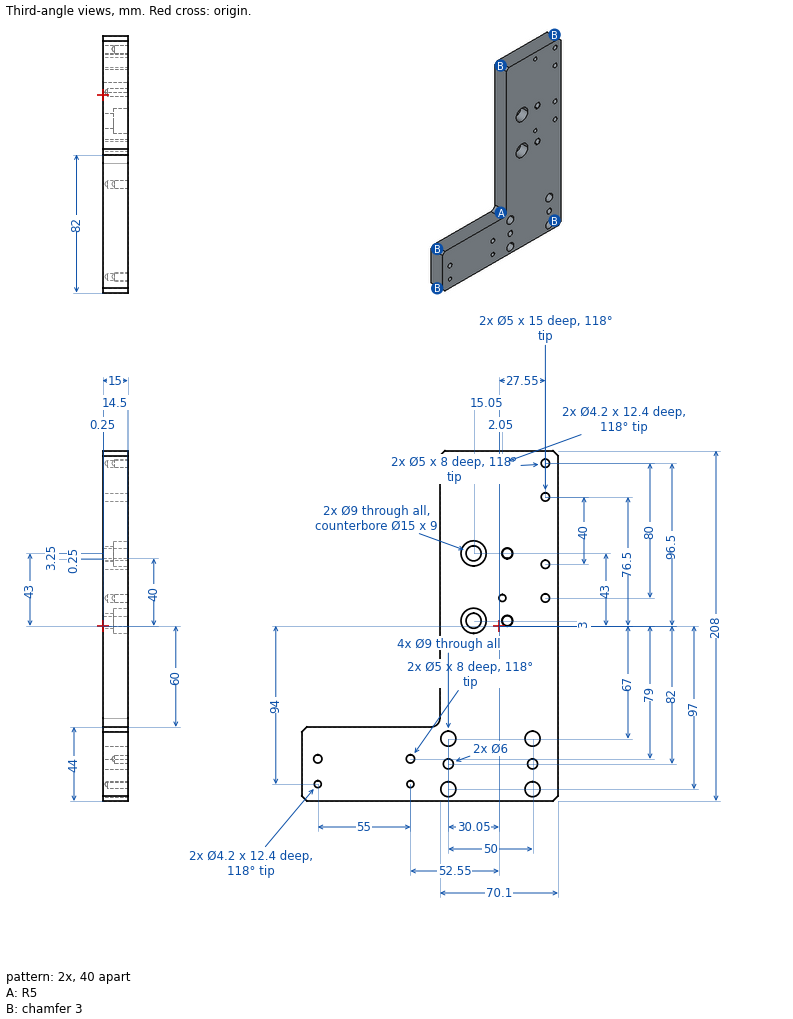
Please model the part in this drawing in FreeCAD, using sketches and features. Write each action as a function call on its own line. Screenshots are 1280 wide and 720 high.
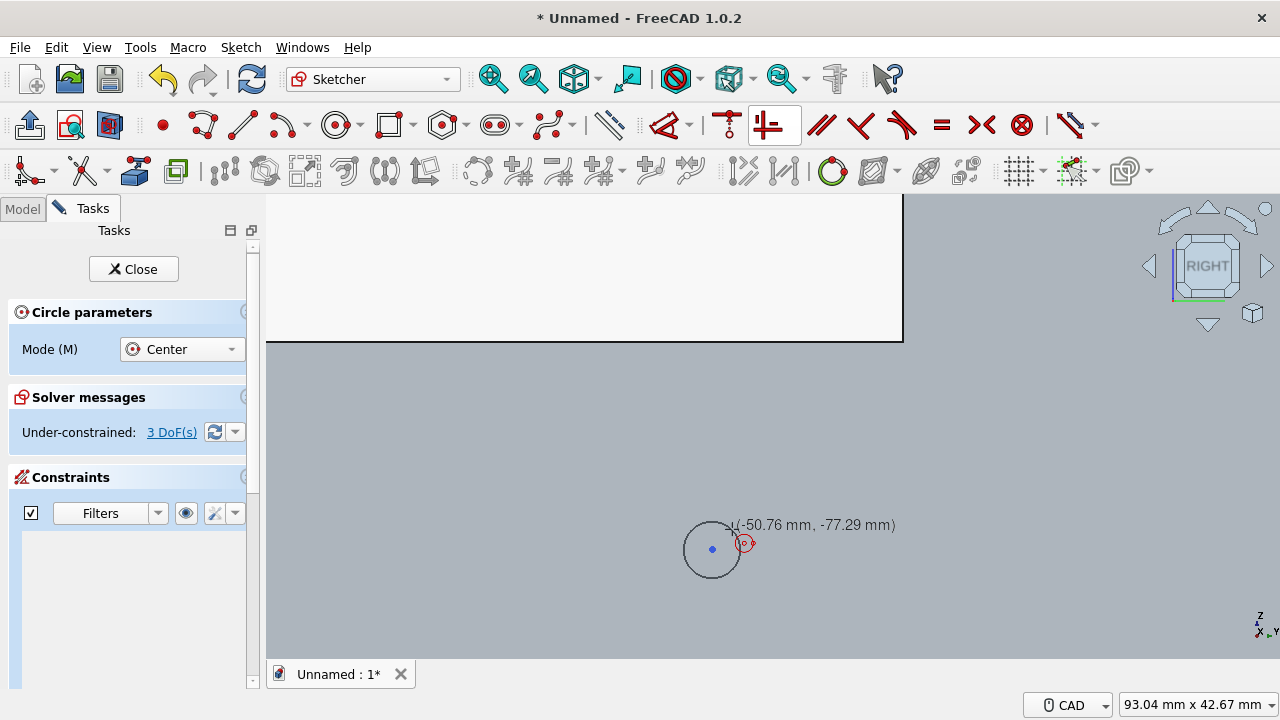
scroll(713, 554, down, 6)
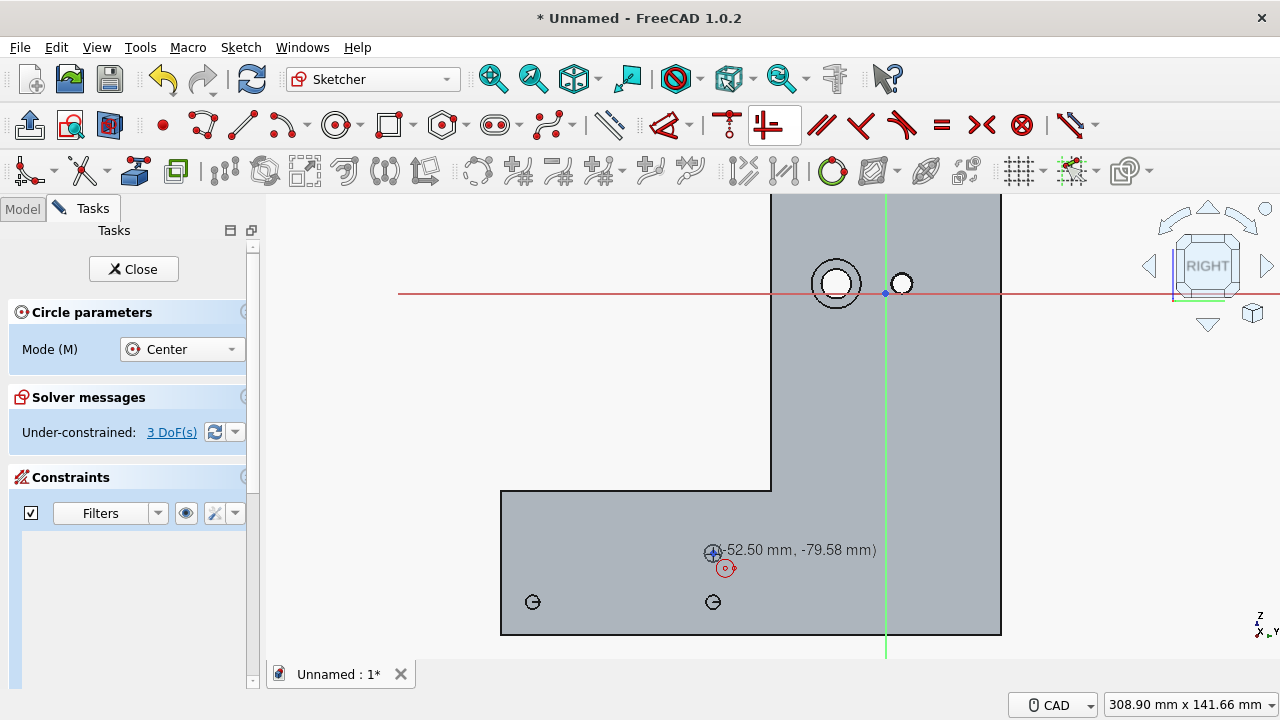
scroll(533, 553, up, 6)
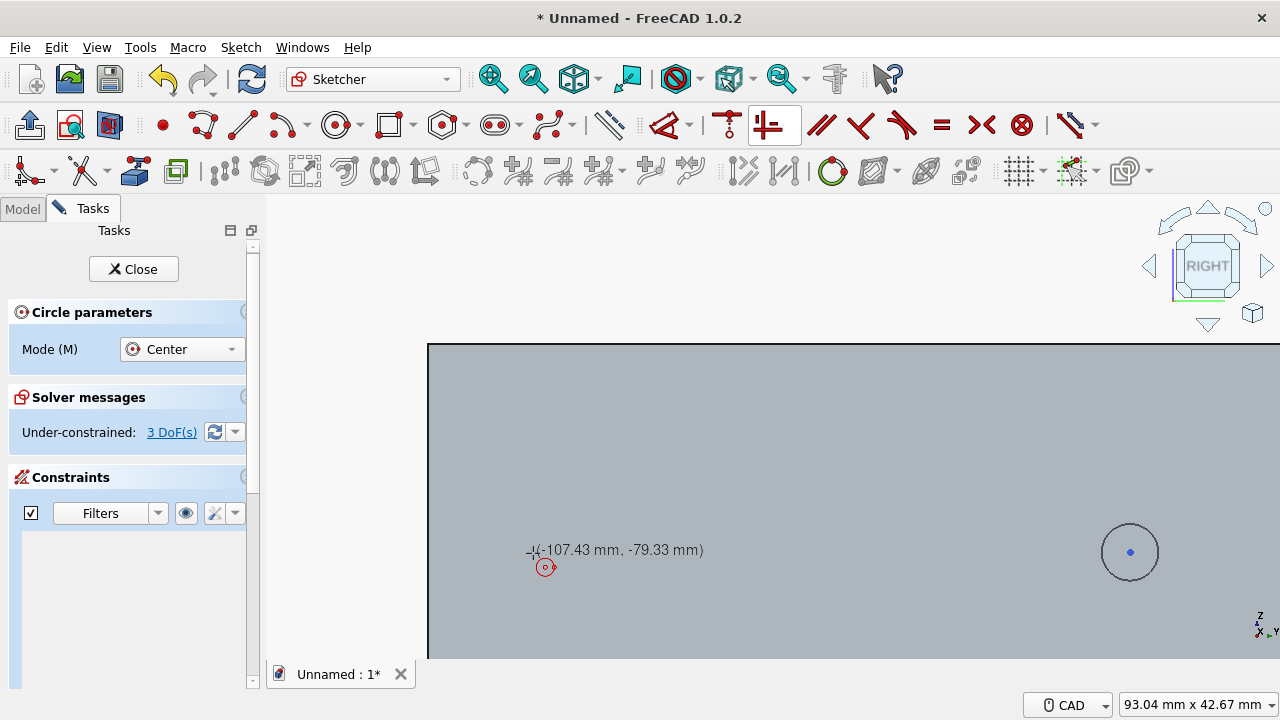
click(531, 551)
click(550, 532)
key(Escape)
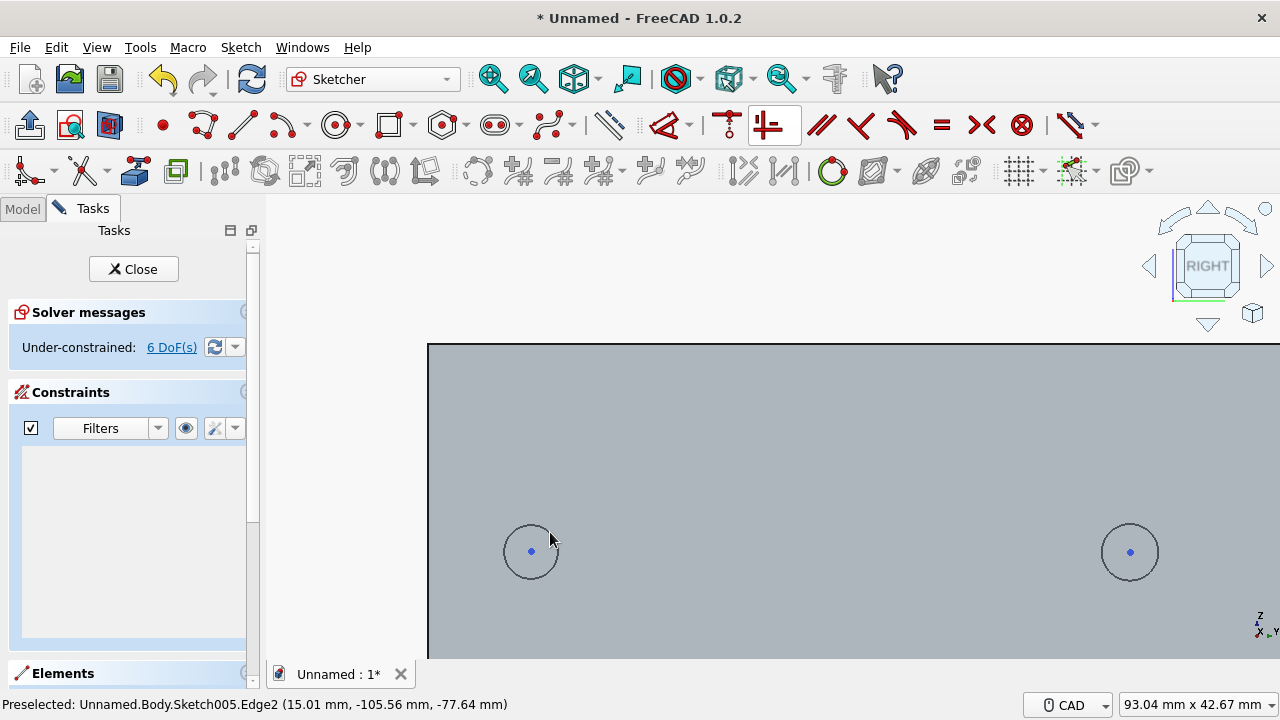
click(1110, 532)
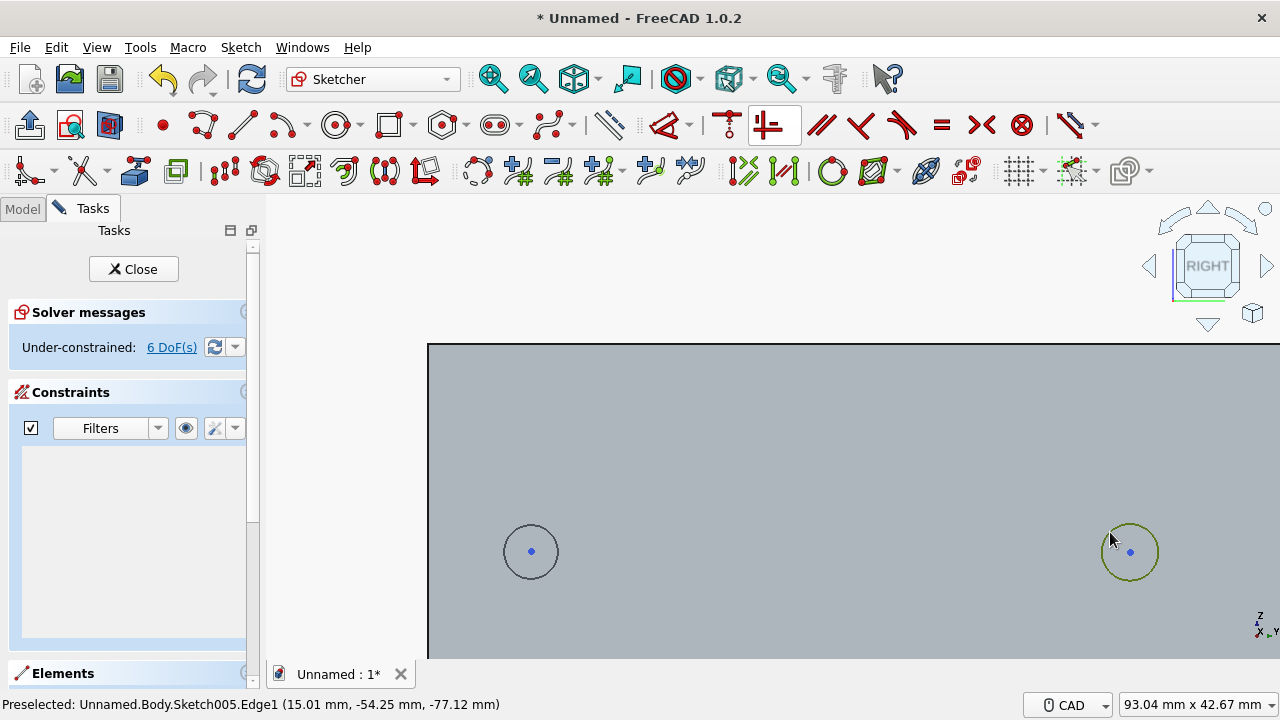
click(550, 533)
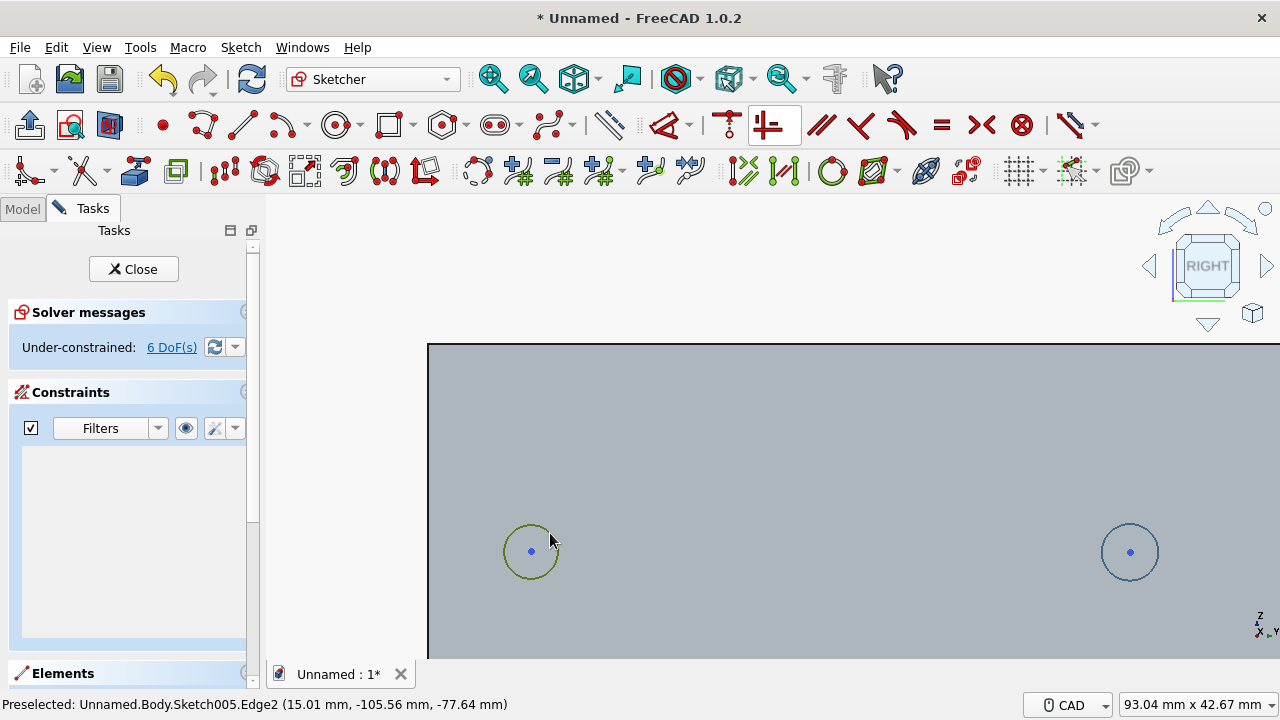
click(942, 126)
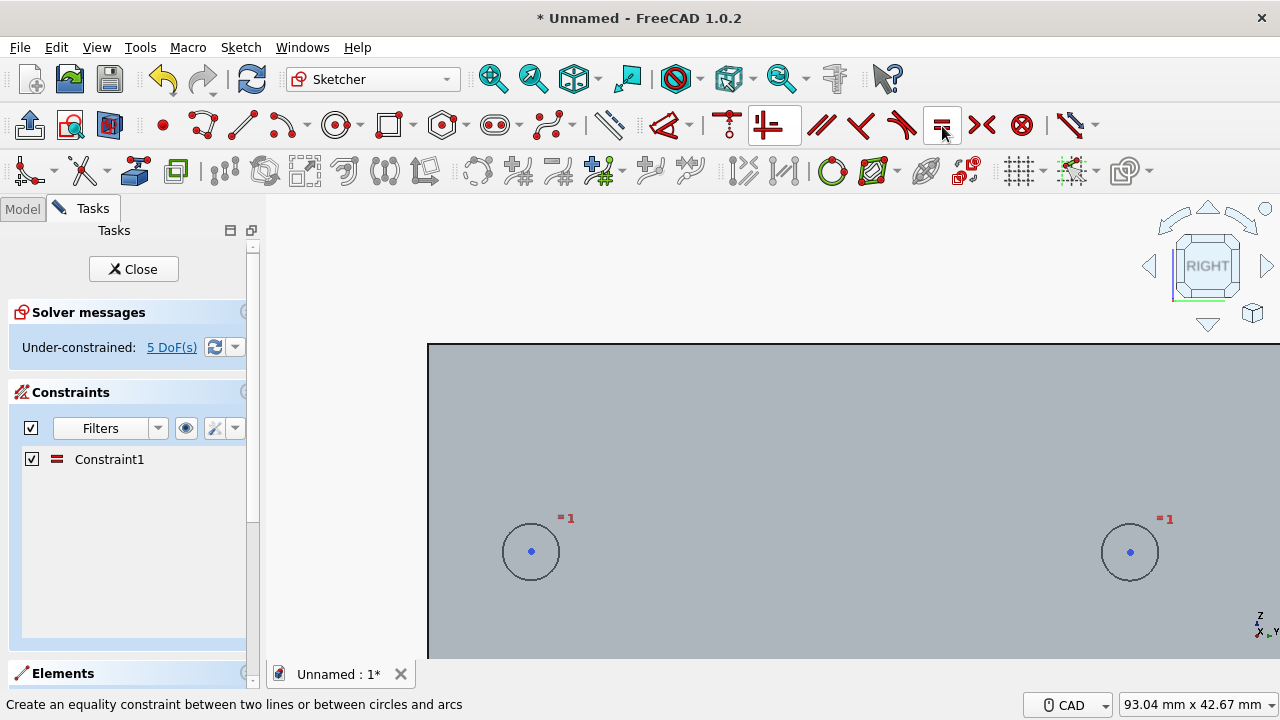
scroll(533, 553, down, 6)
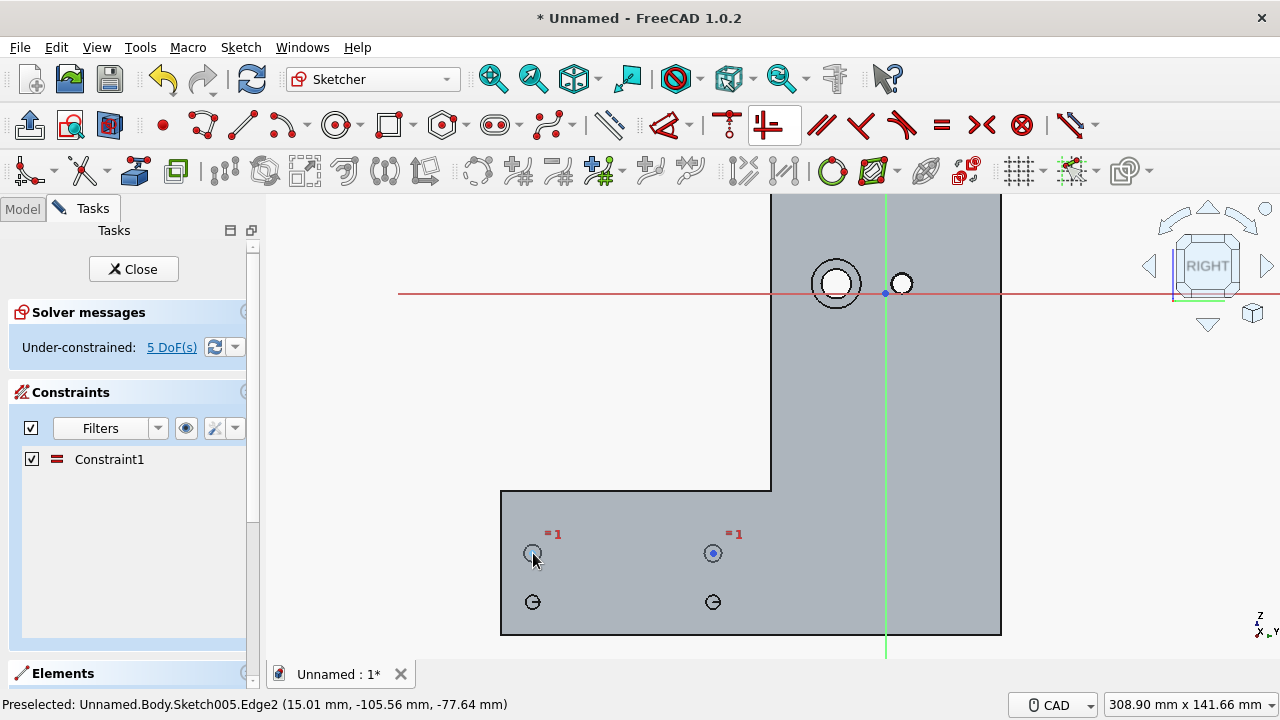
click(713, 553)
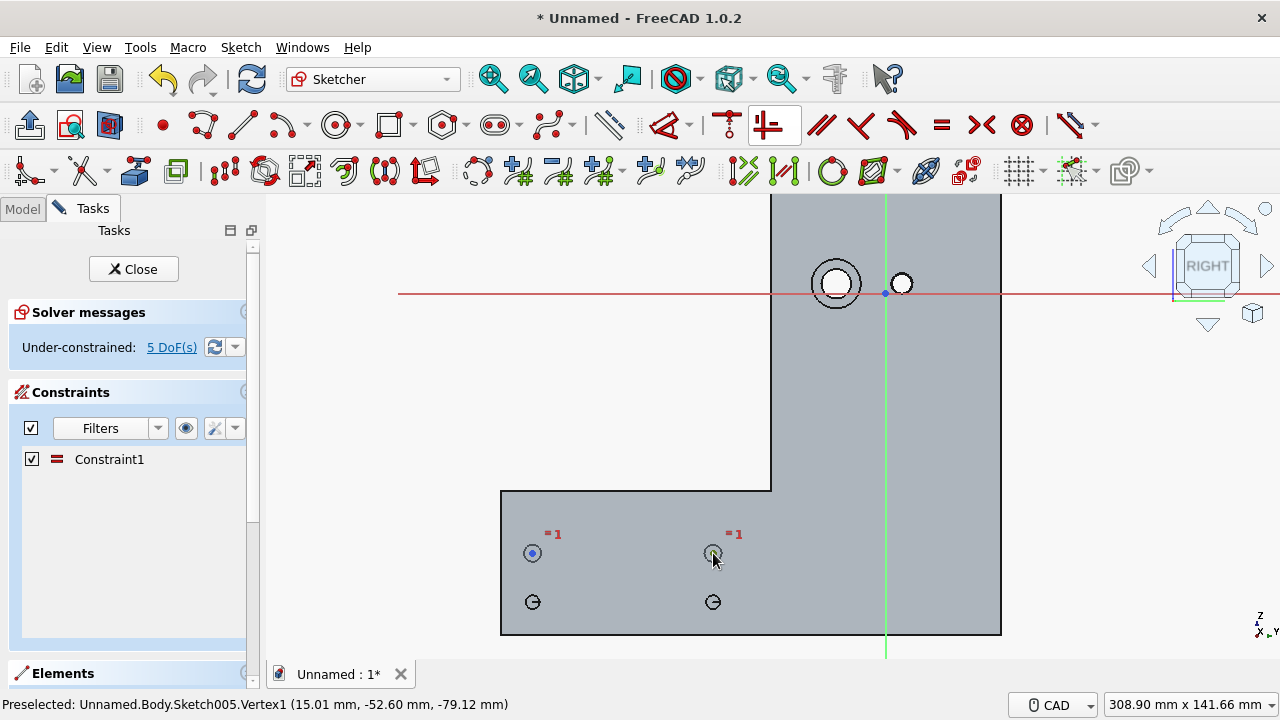
click(533, 553)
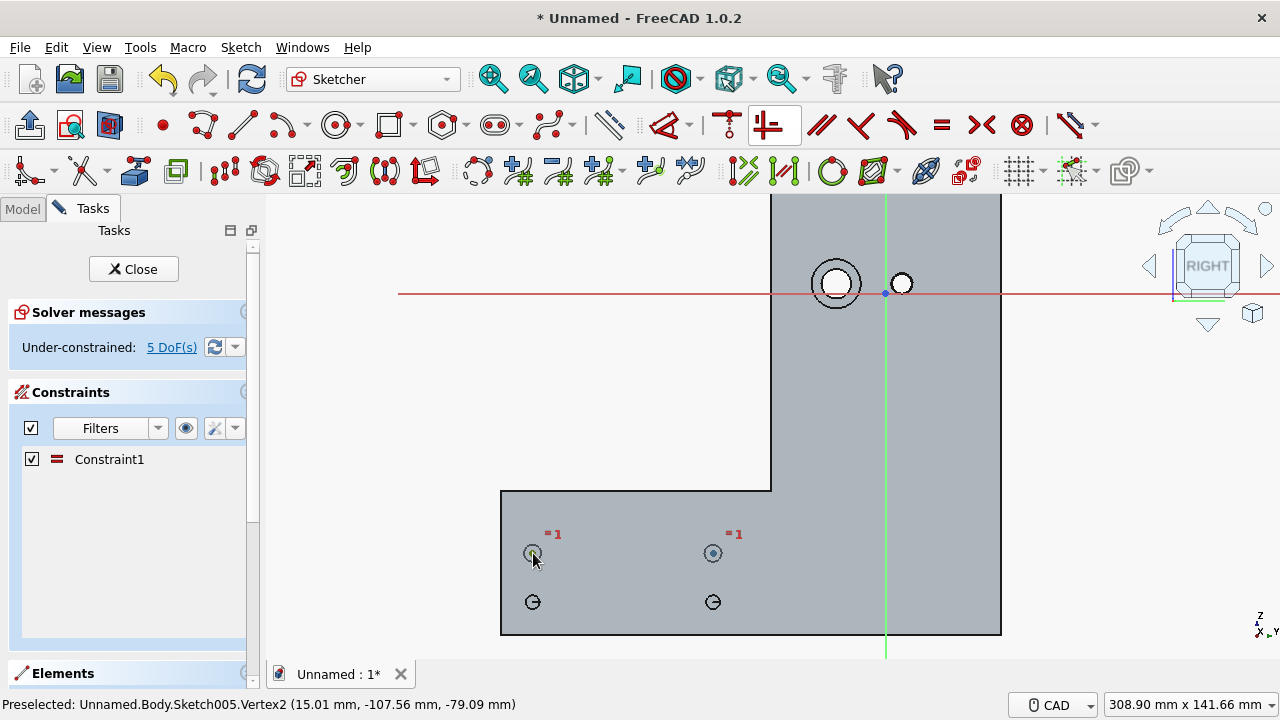
key(h)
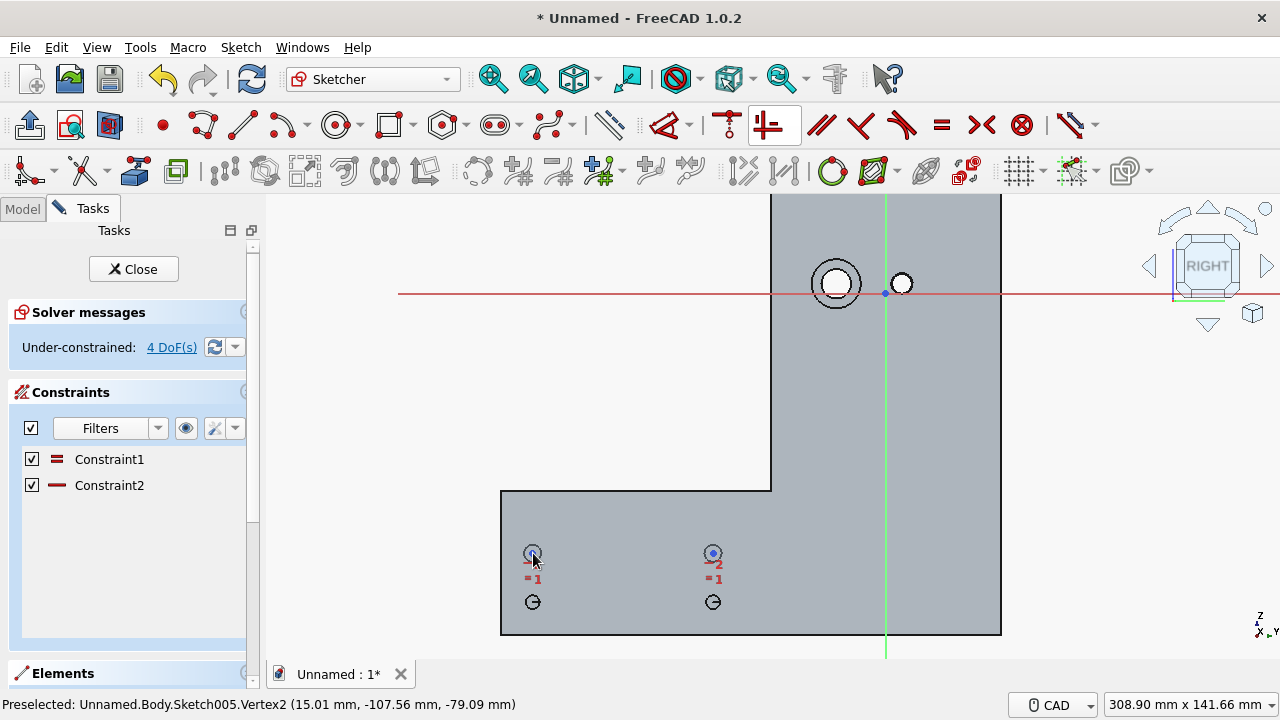
click(664, 126)